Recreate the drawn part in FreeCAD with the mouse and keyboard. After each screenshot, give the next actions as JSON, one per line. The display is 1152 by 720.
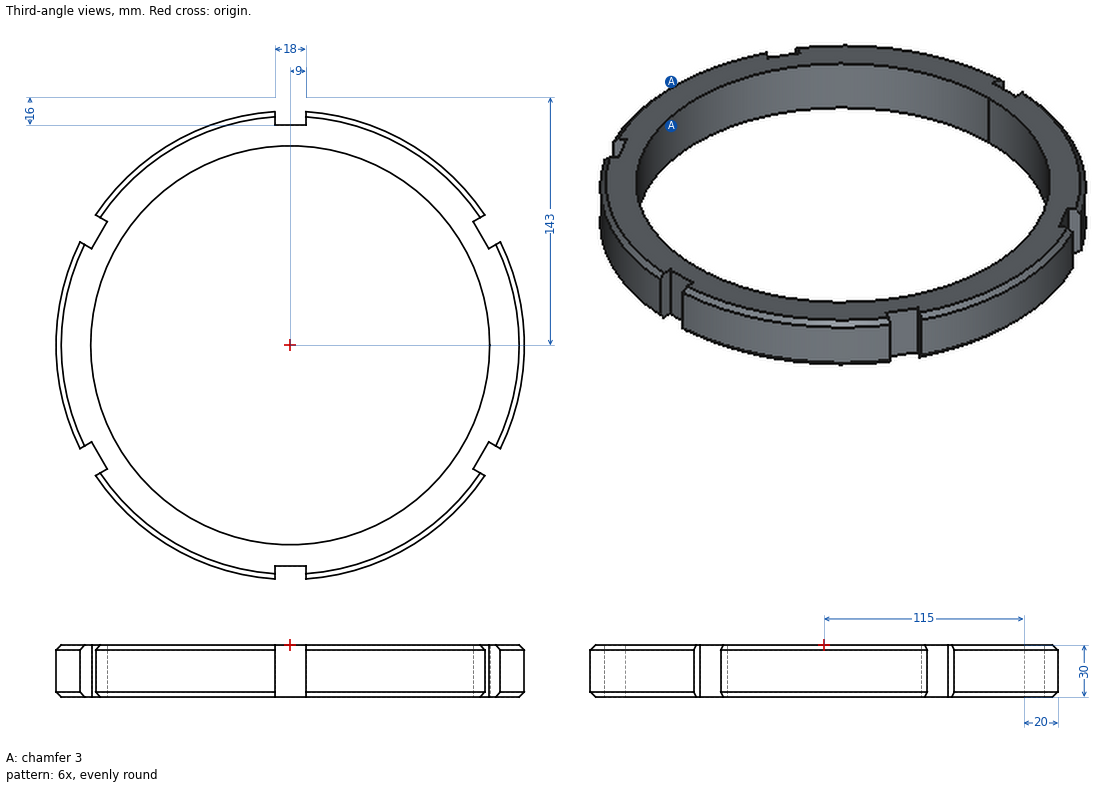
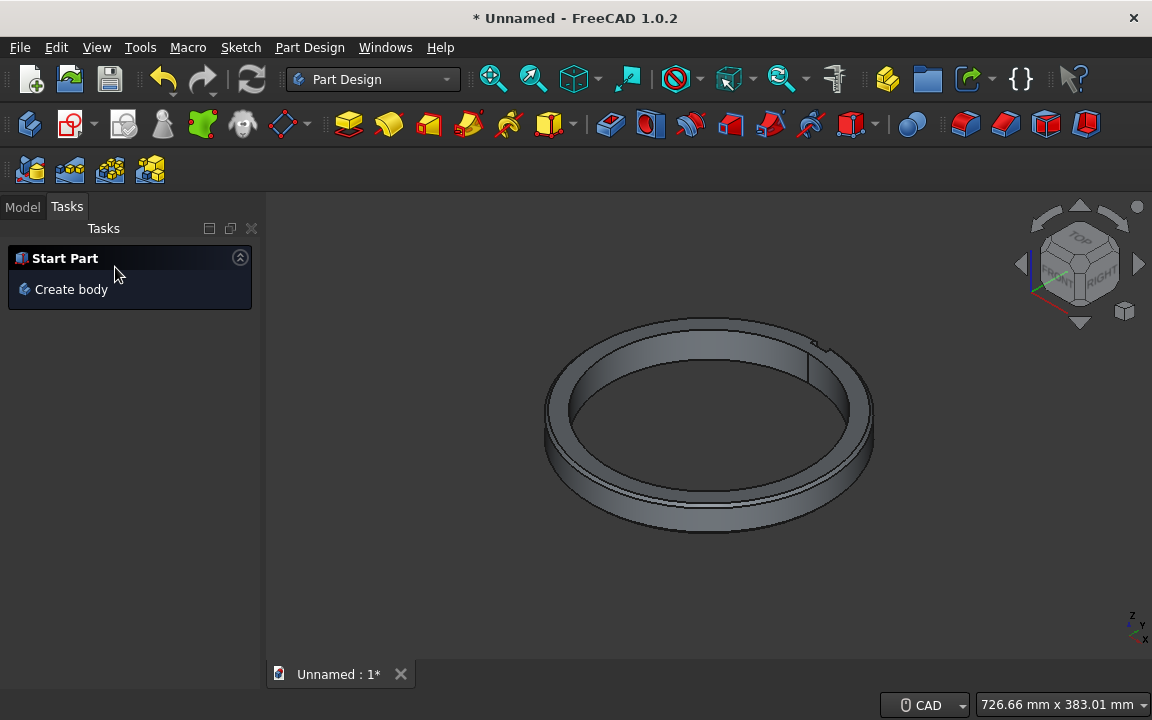
{"action": "left_click", "coordinate": [23, 206]}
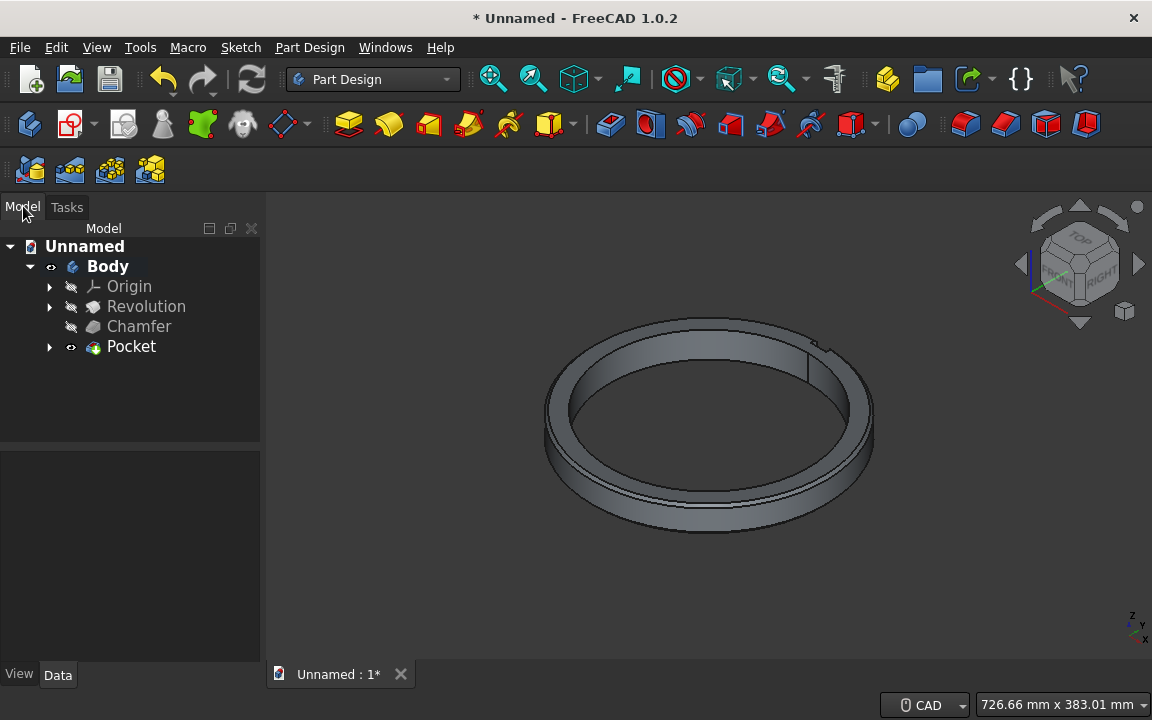
{"action": "left_click", "coordinate": [116, 347]}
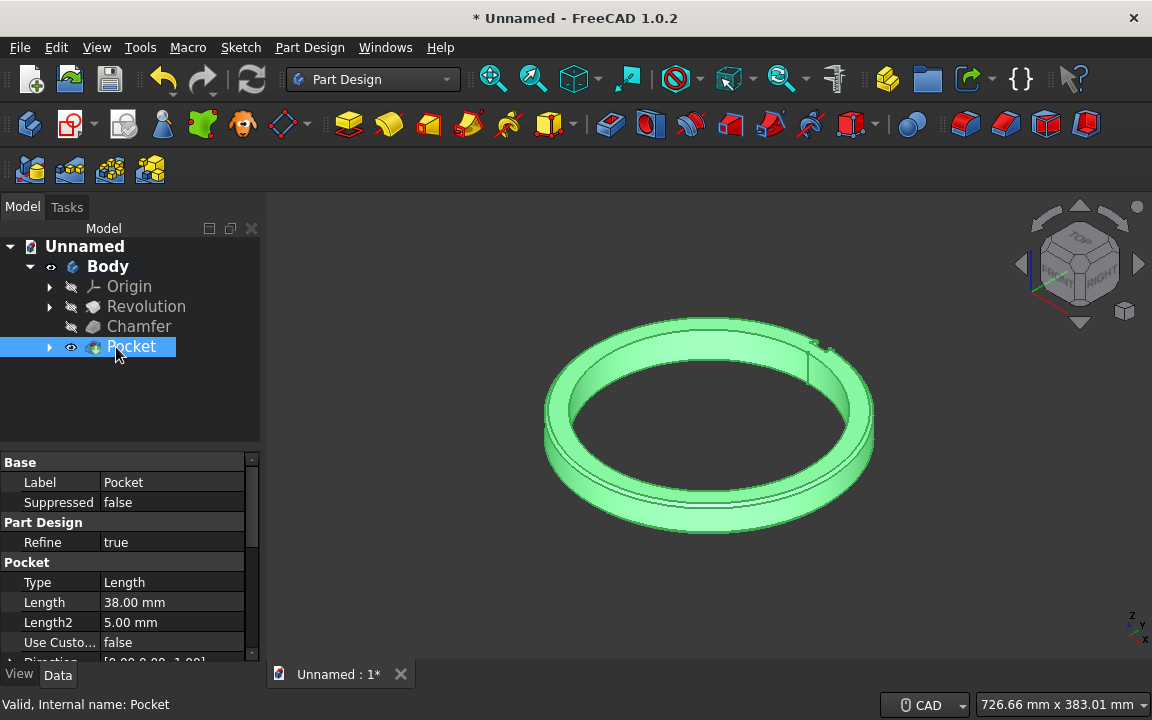
{"action": "left_click", "coordinate": [110, 170]}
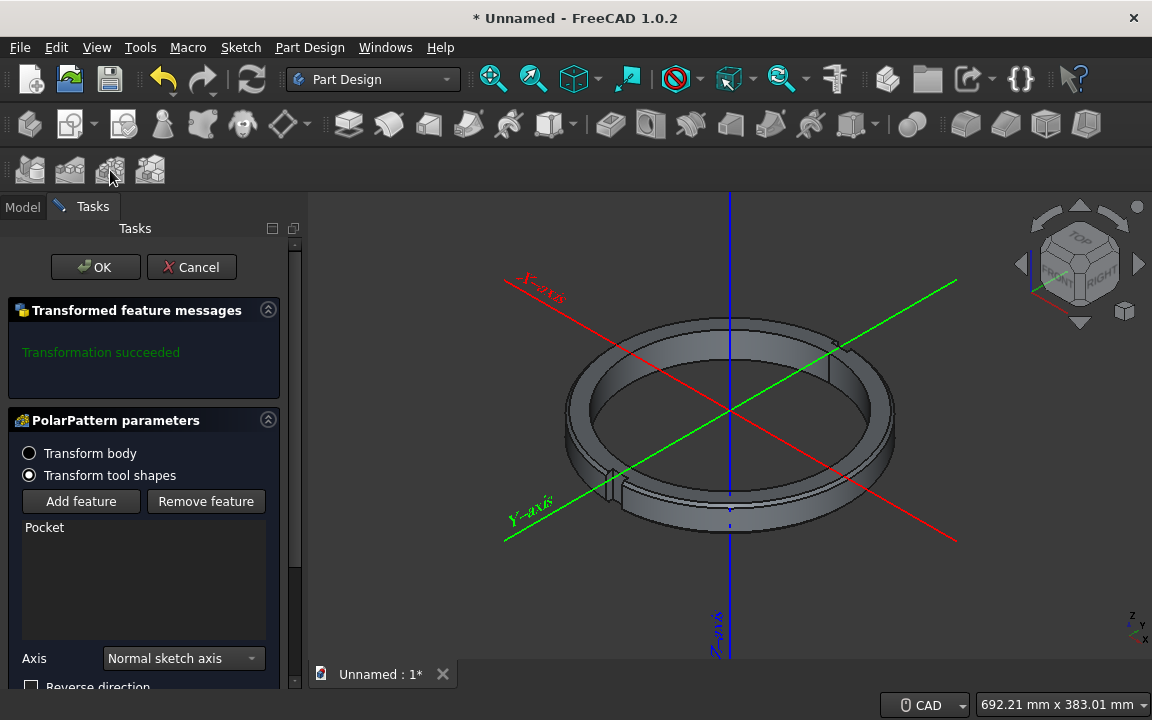
{"action": "left_click", "coordinate": [184, 658]}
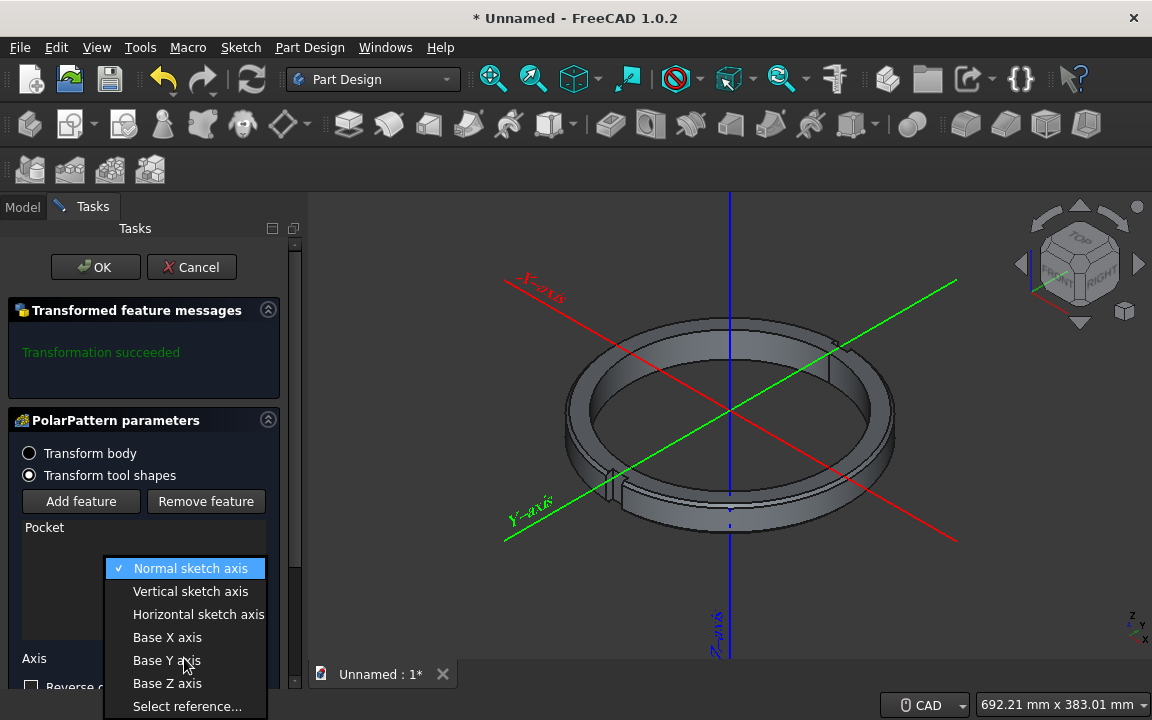
{"action": "left_click", "coordinate": [184, 684]}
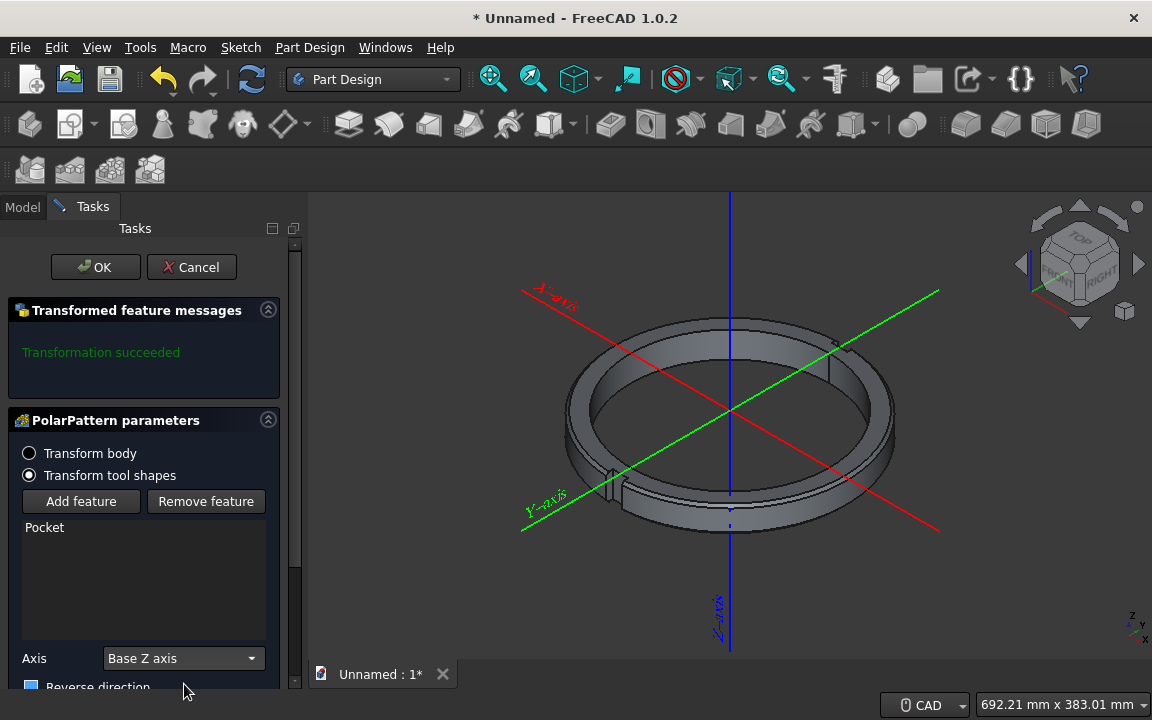
{"action": "scroll", "coordinate": [295, 463], "scroll_direction": "down", "scroll_amount": 3}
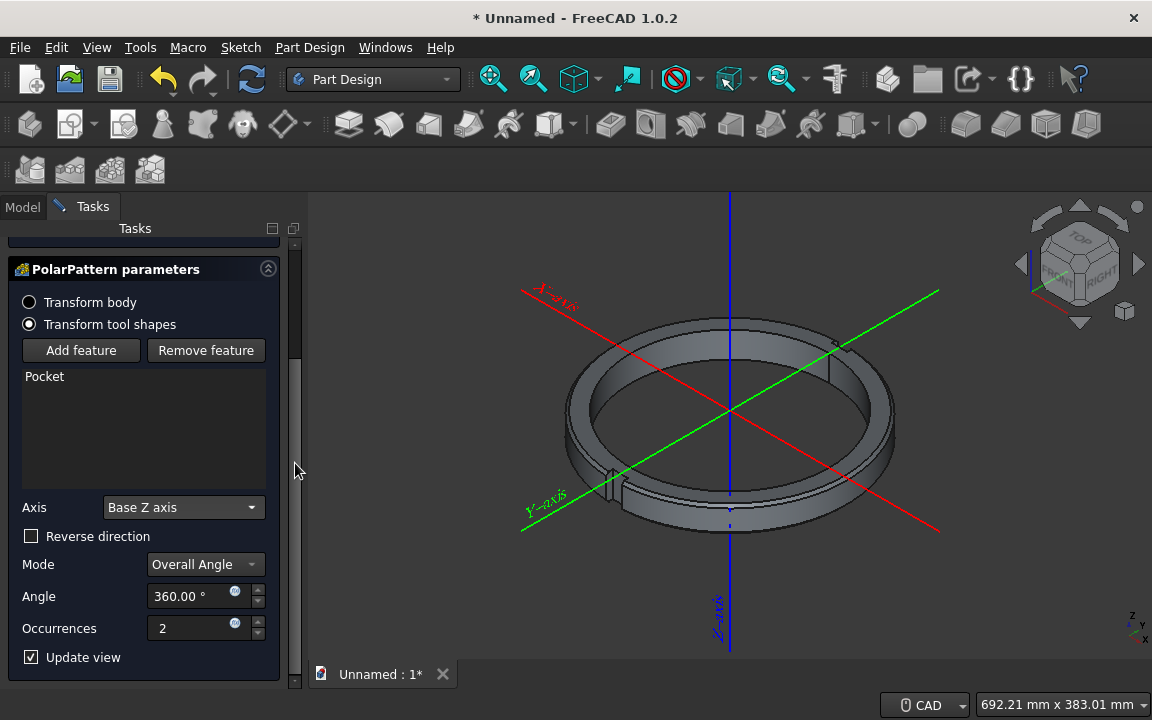
{"action": "triple_click", "coordinate": [198, 628]}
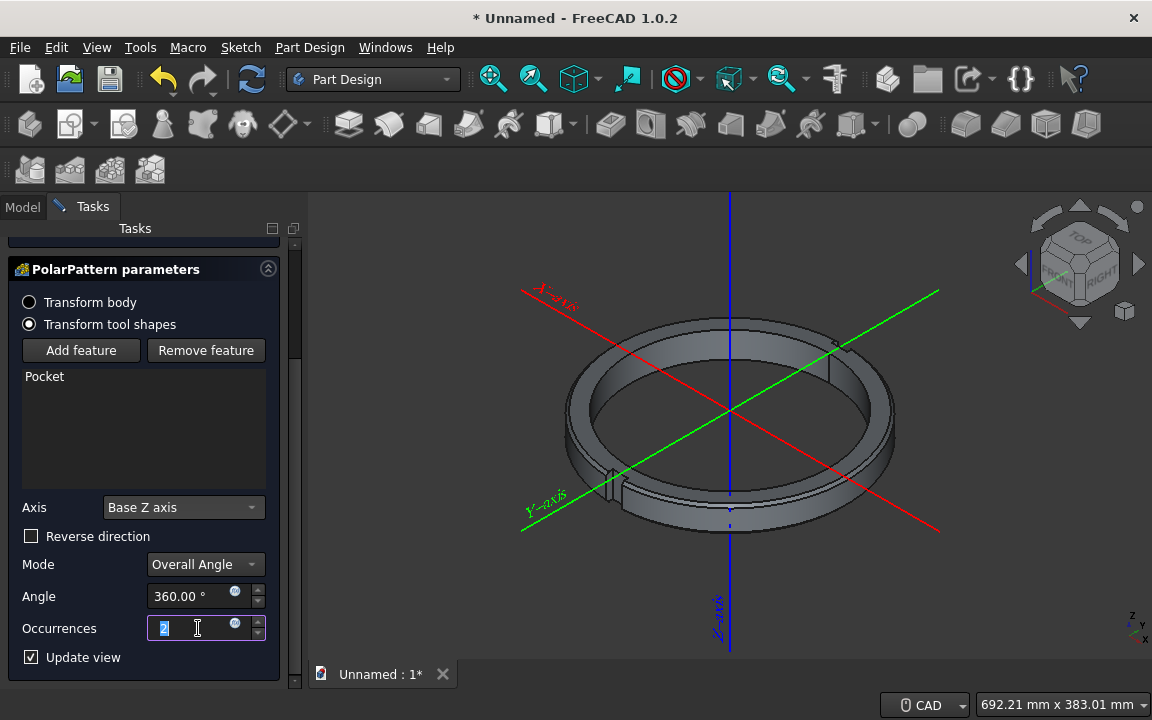
{"action": "type", "text": "6"}
{"action": "key", "text": "Tab"}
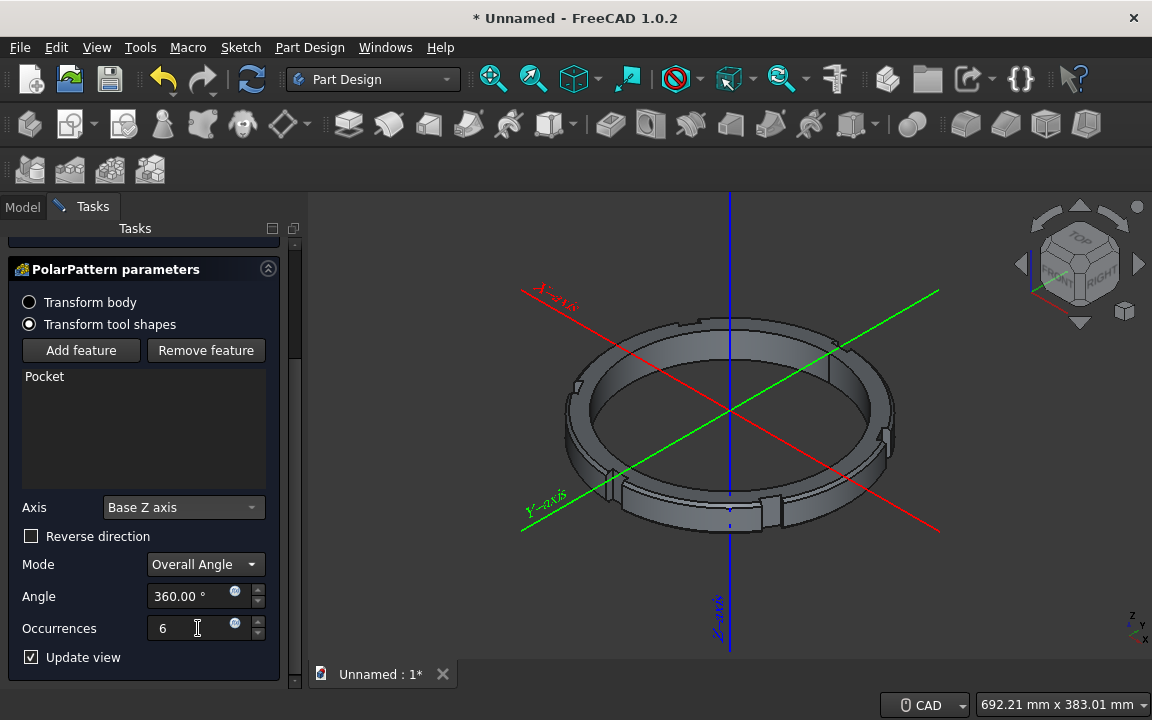
{"action": "scroll", "coordinate": [295, 463], "scroll_direction": "up", "scroll_amount": 4}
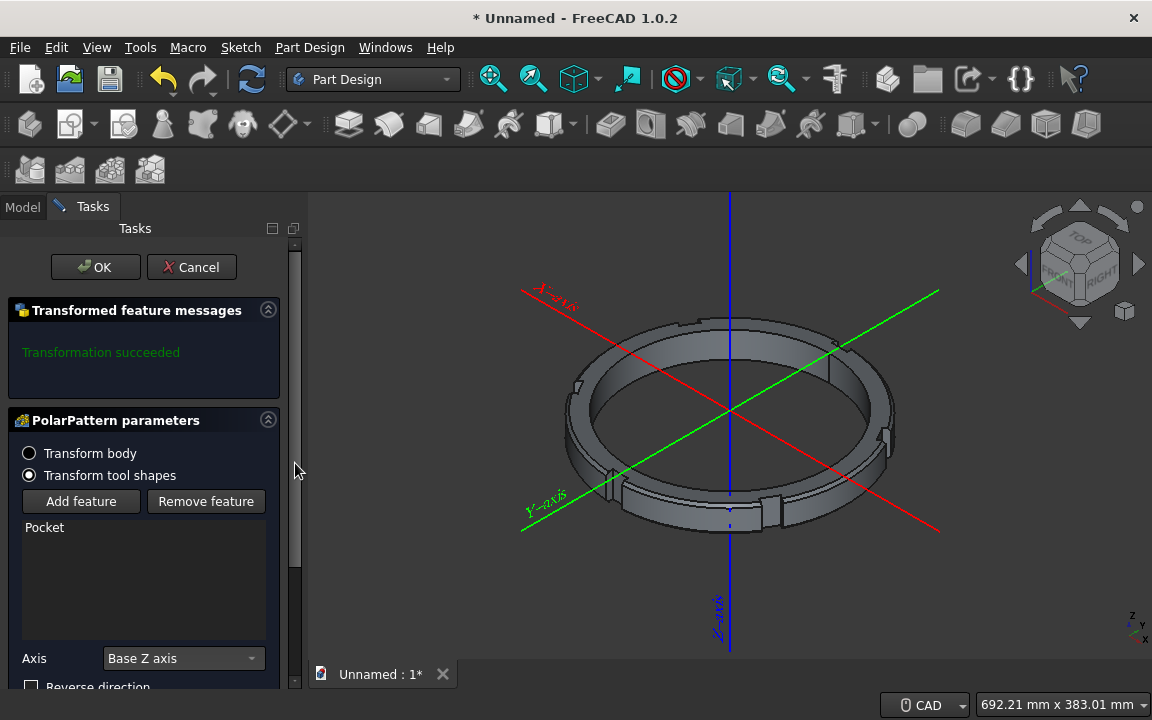
{"action": "left_click", "coordinate": [96, 267]}